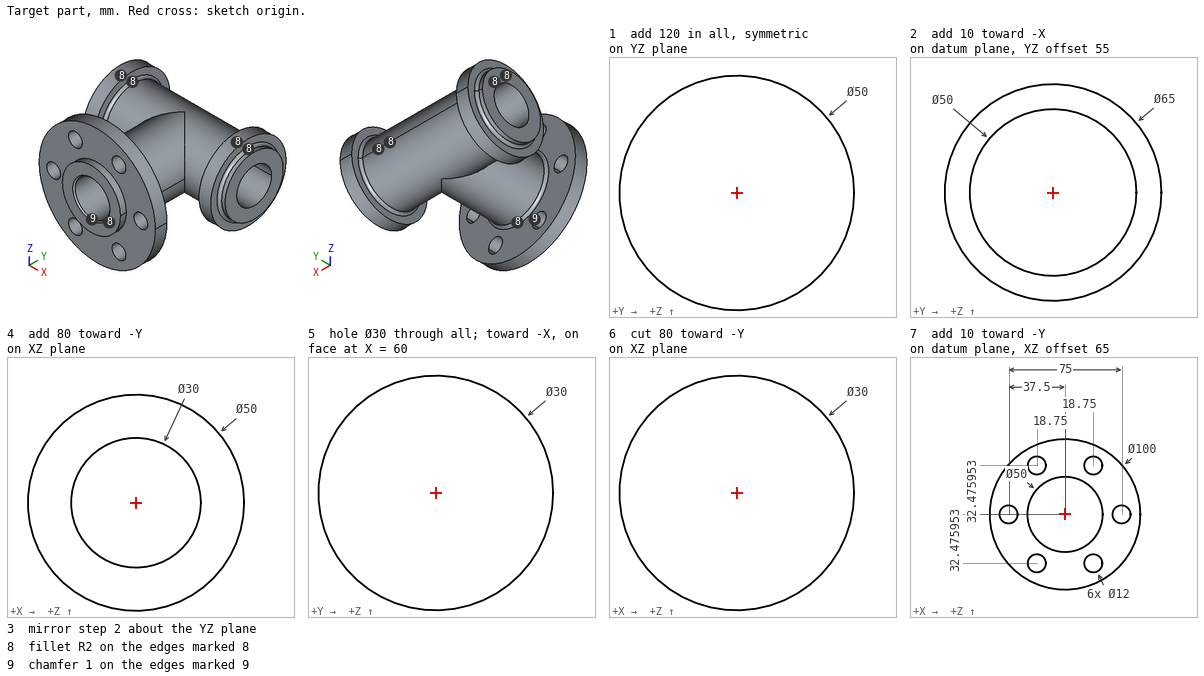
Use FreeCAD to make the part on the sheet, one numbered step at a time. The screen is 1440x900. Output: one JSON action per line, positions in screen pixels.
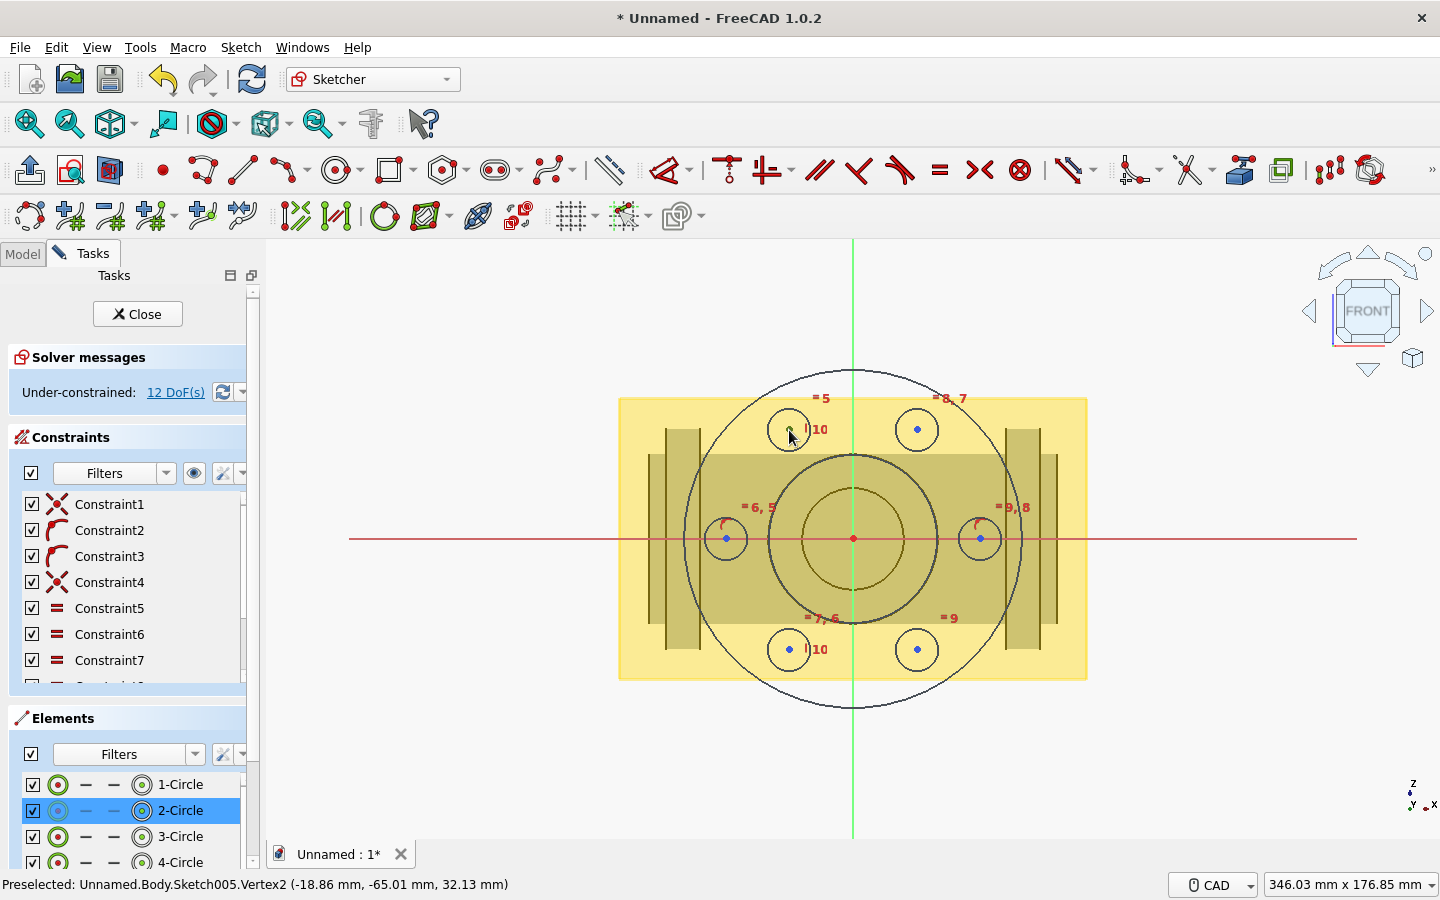
{"action": "left_click", "coordinate": [917, 430]}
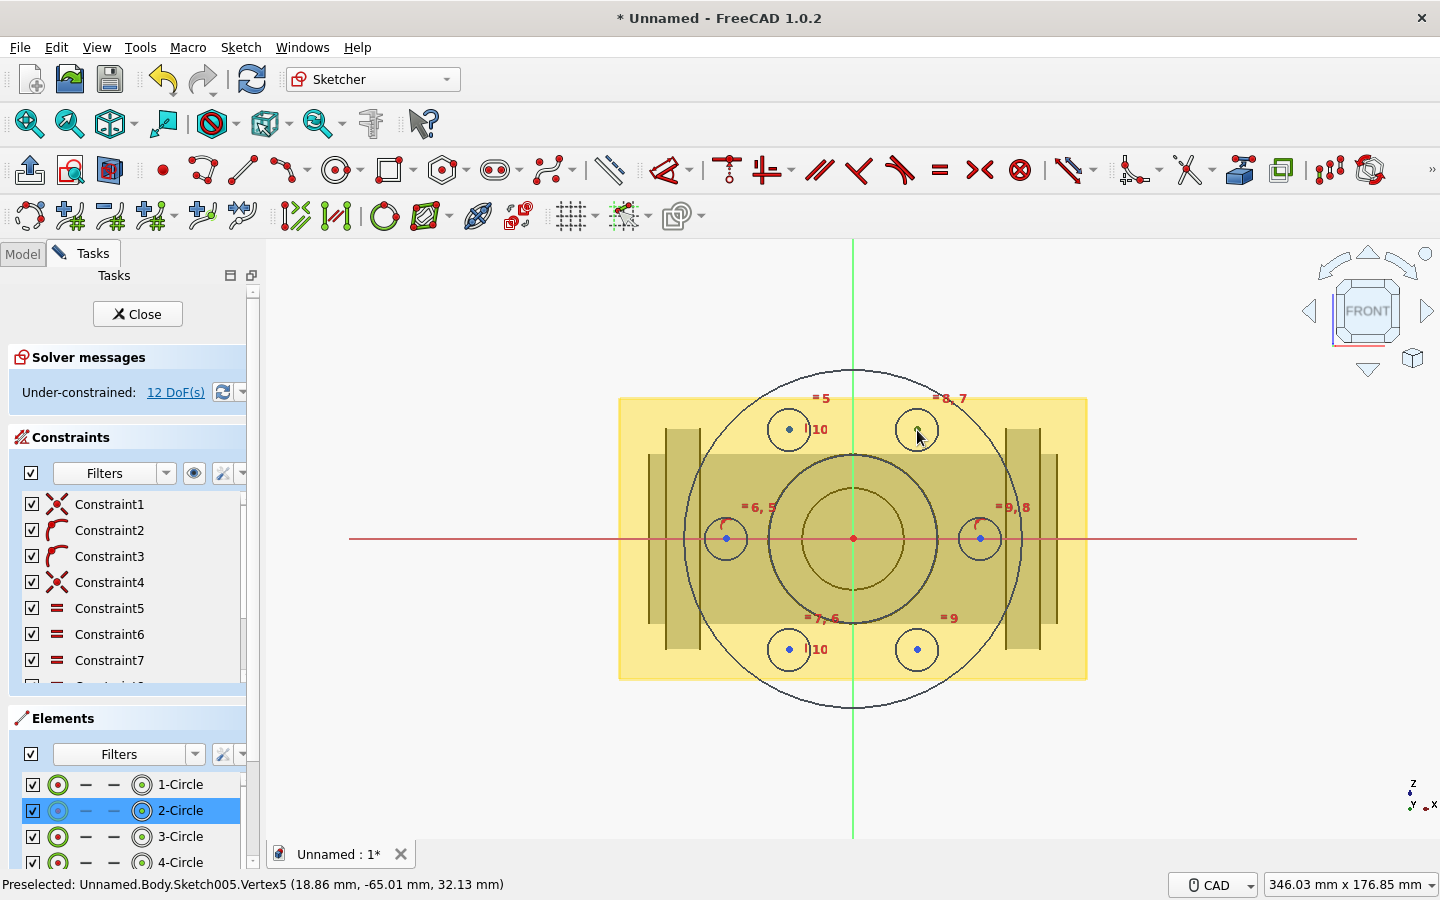
{"action": "left_click", "coordinate": [794, 170]}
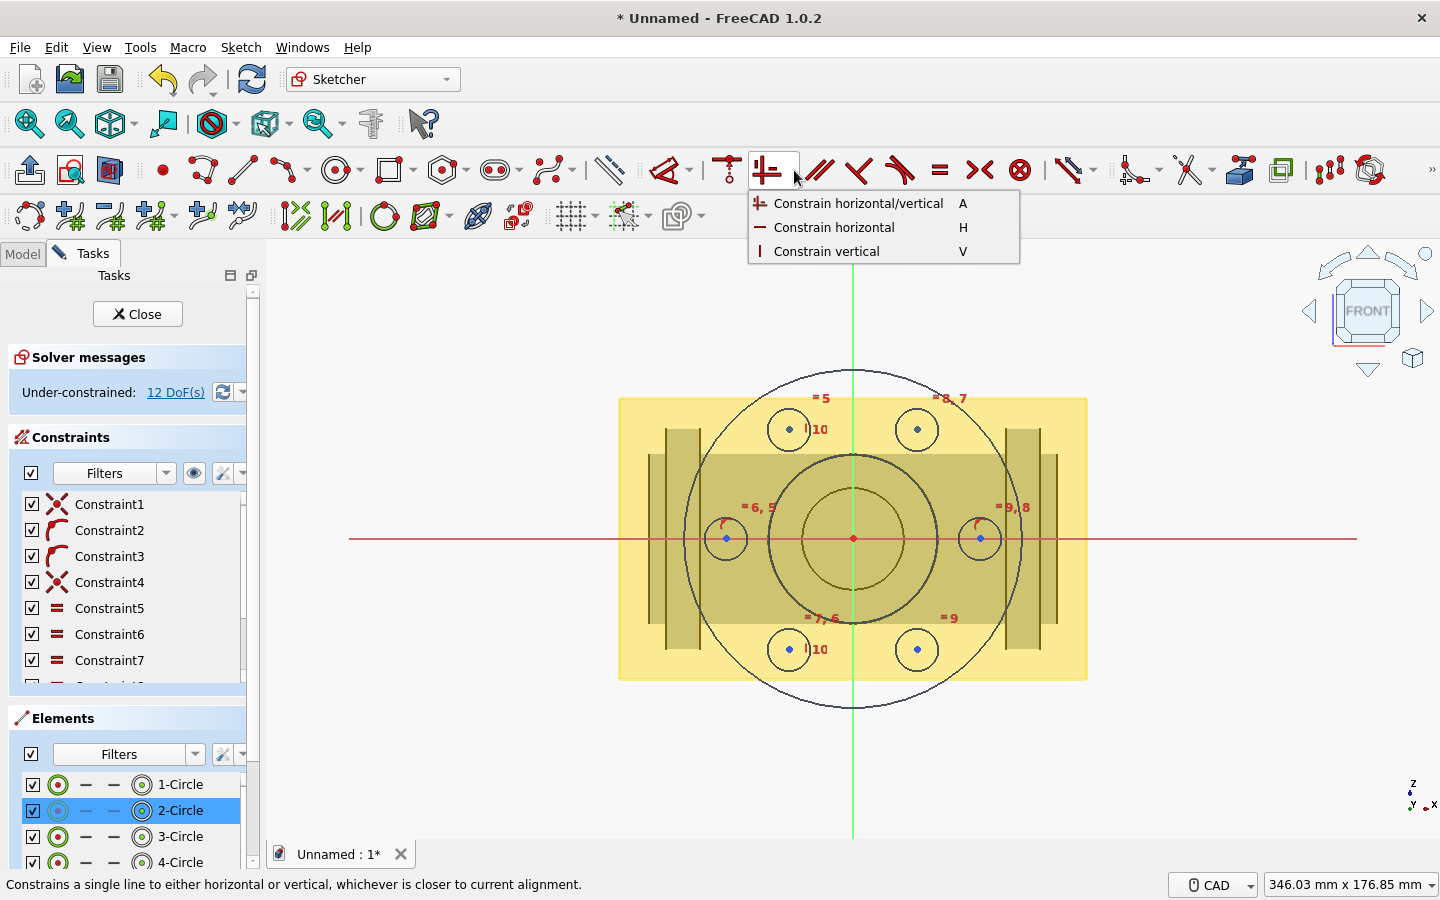
{"action": "left_click", "coordinate": [884, 227]}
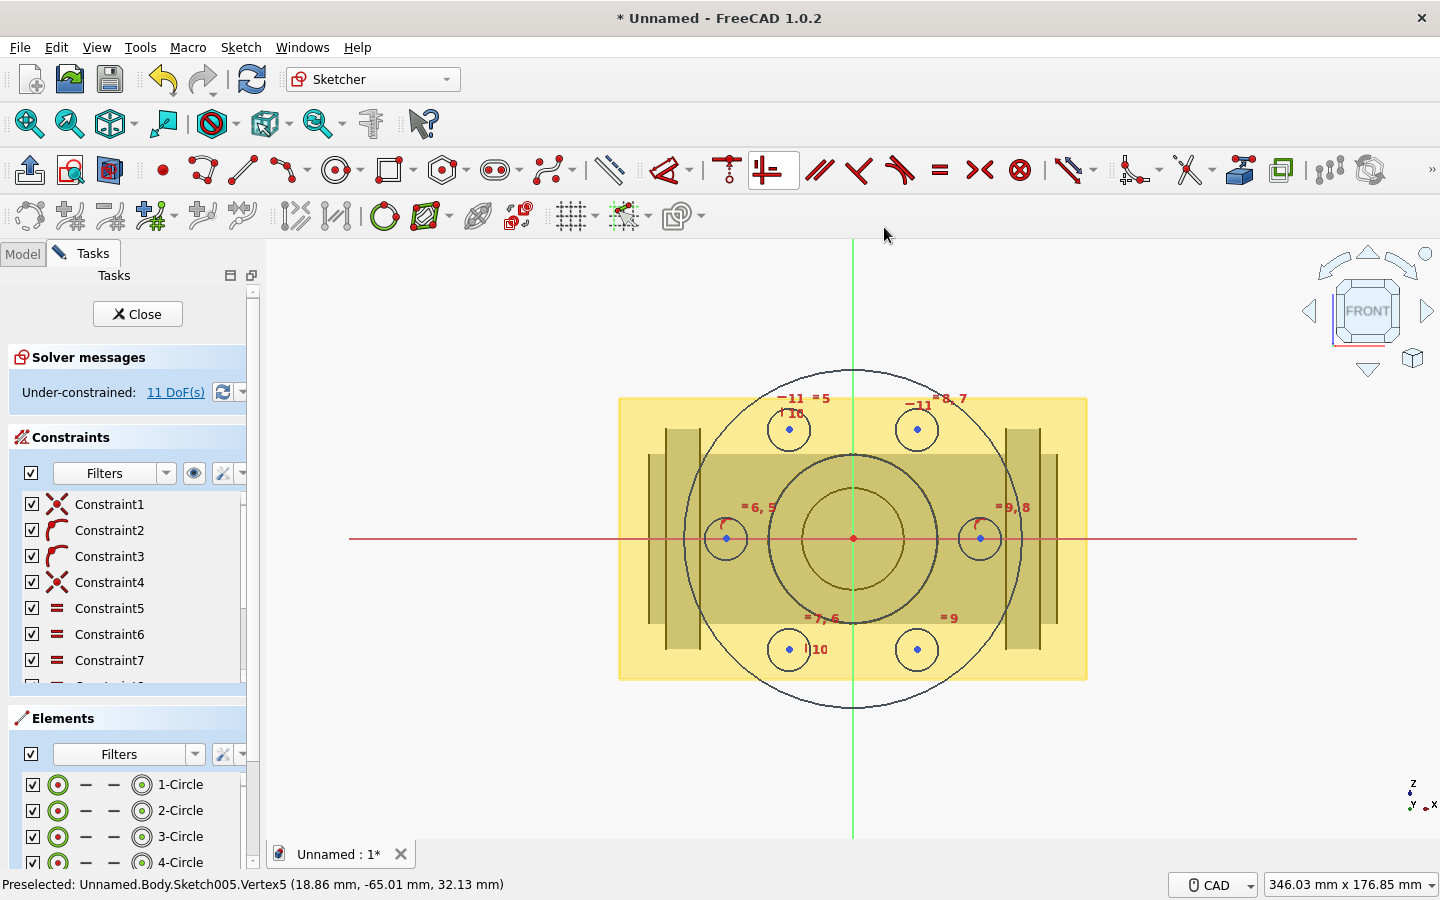
{"action": "left_click", "coordinate": [917, 430]}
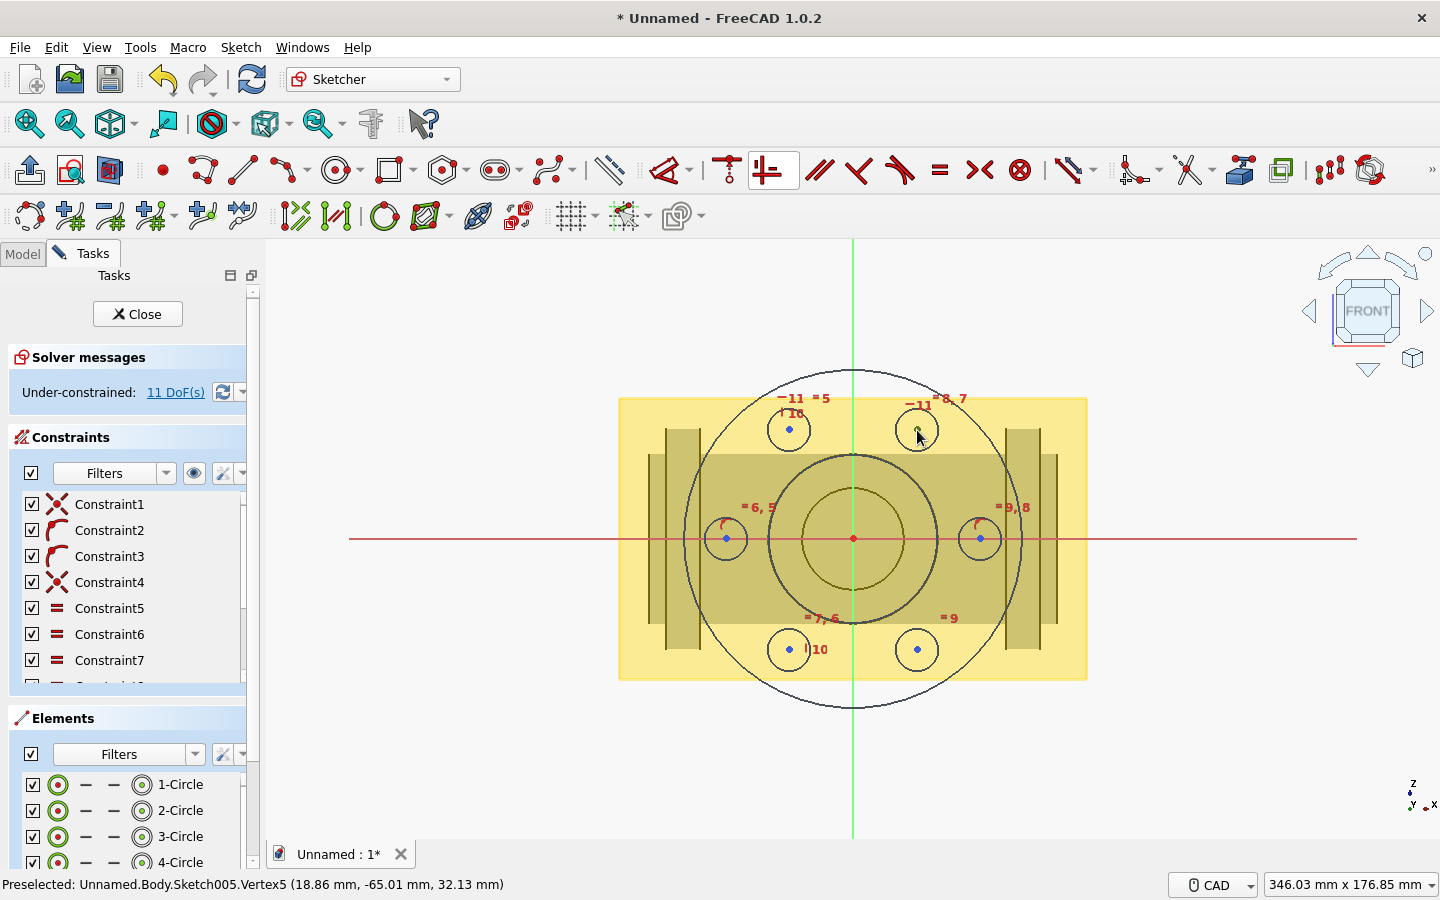
{"action": "left_click", "coordinate": [917, 650]}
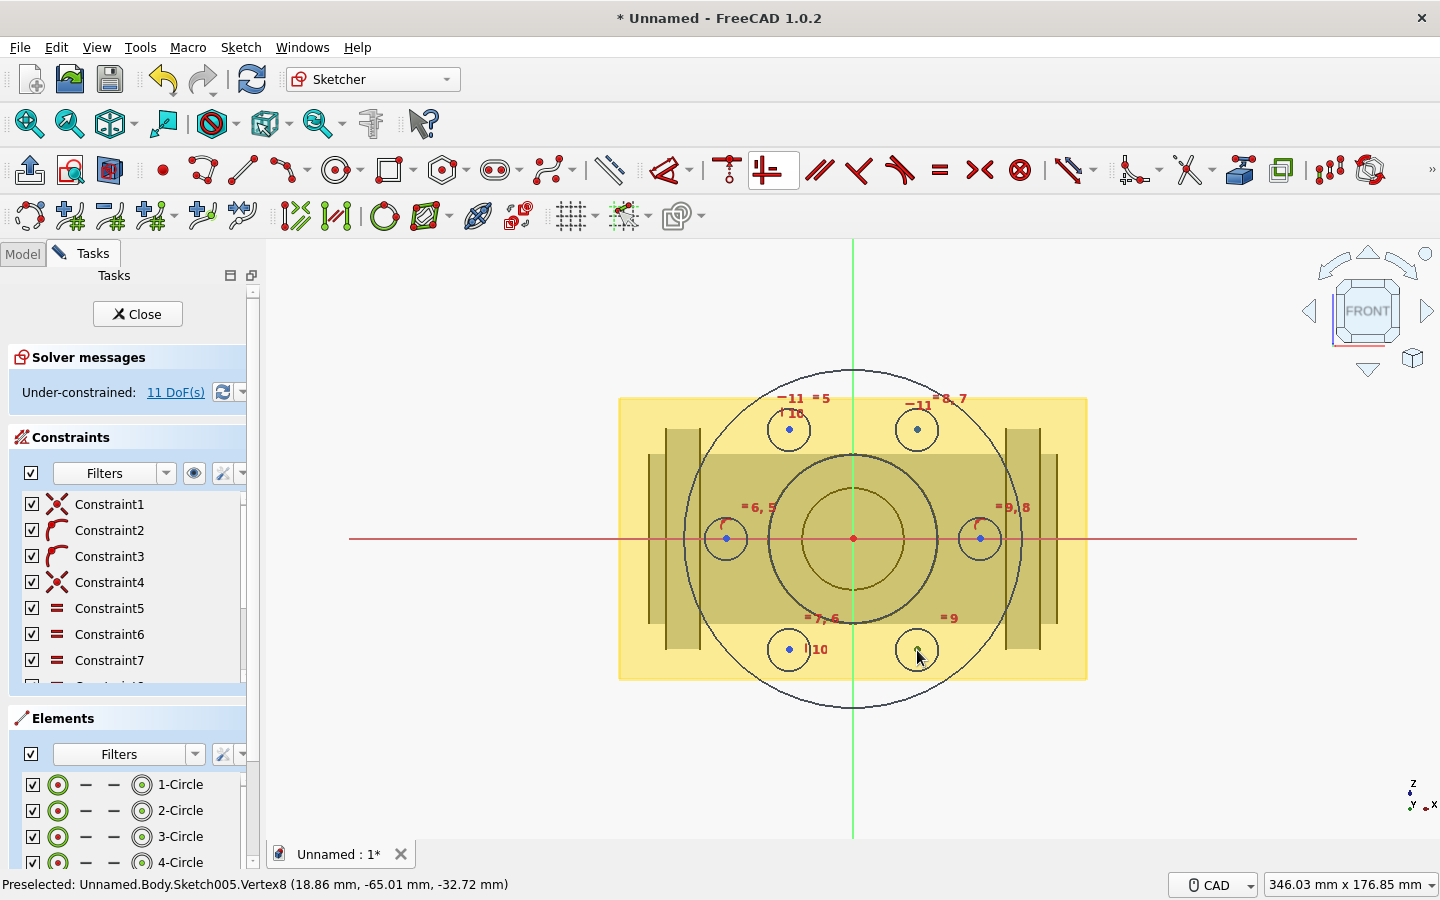
{"action": "key", "text": "v"}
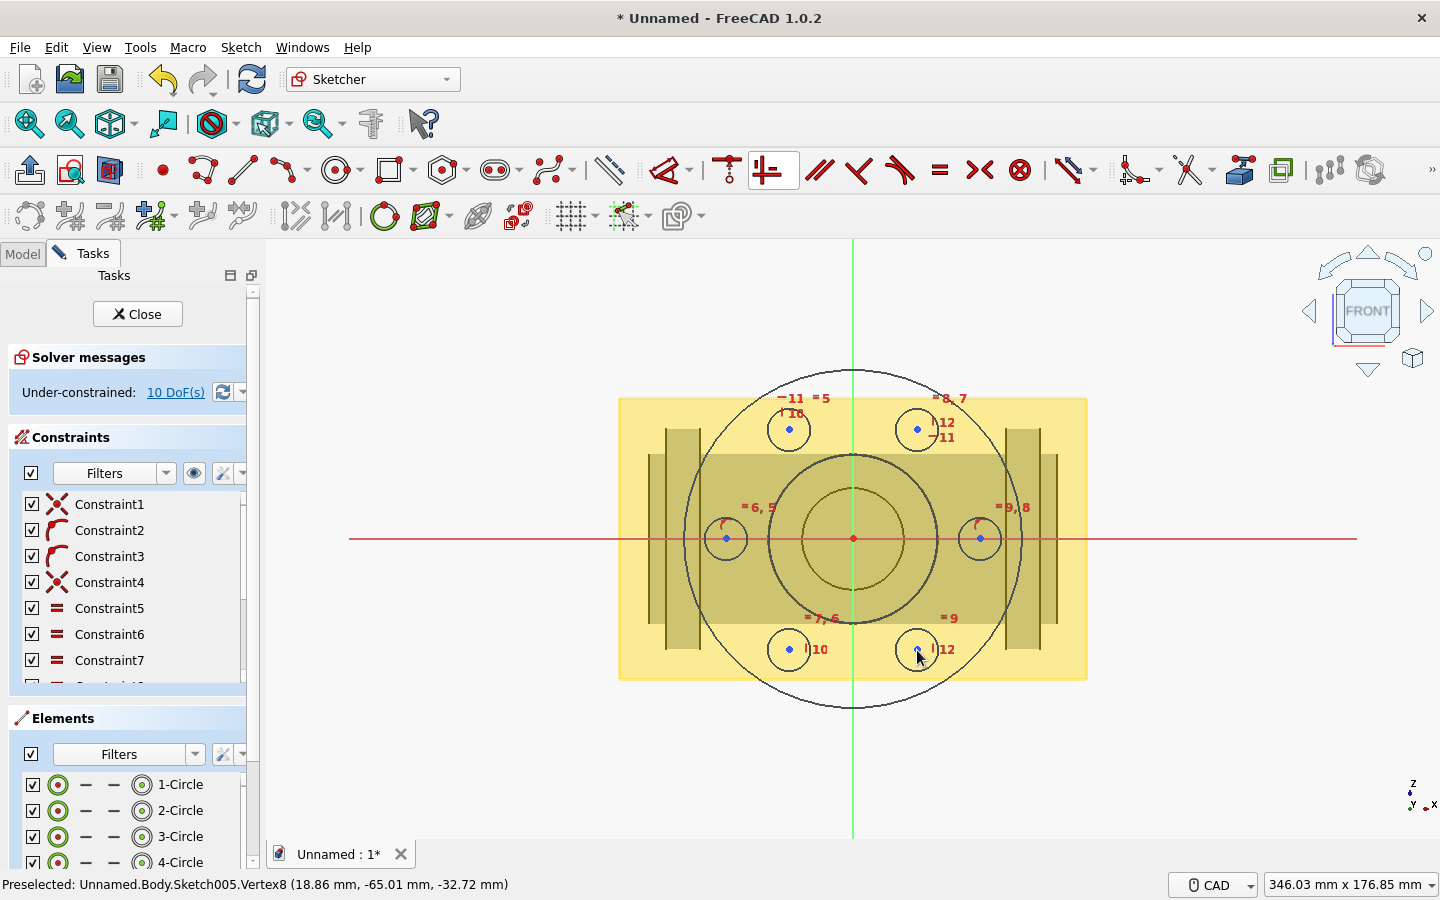
{"action": "left_click", "coordinate": [789, 650]}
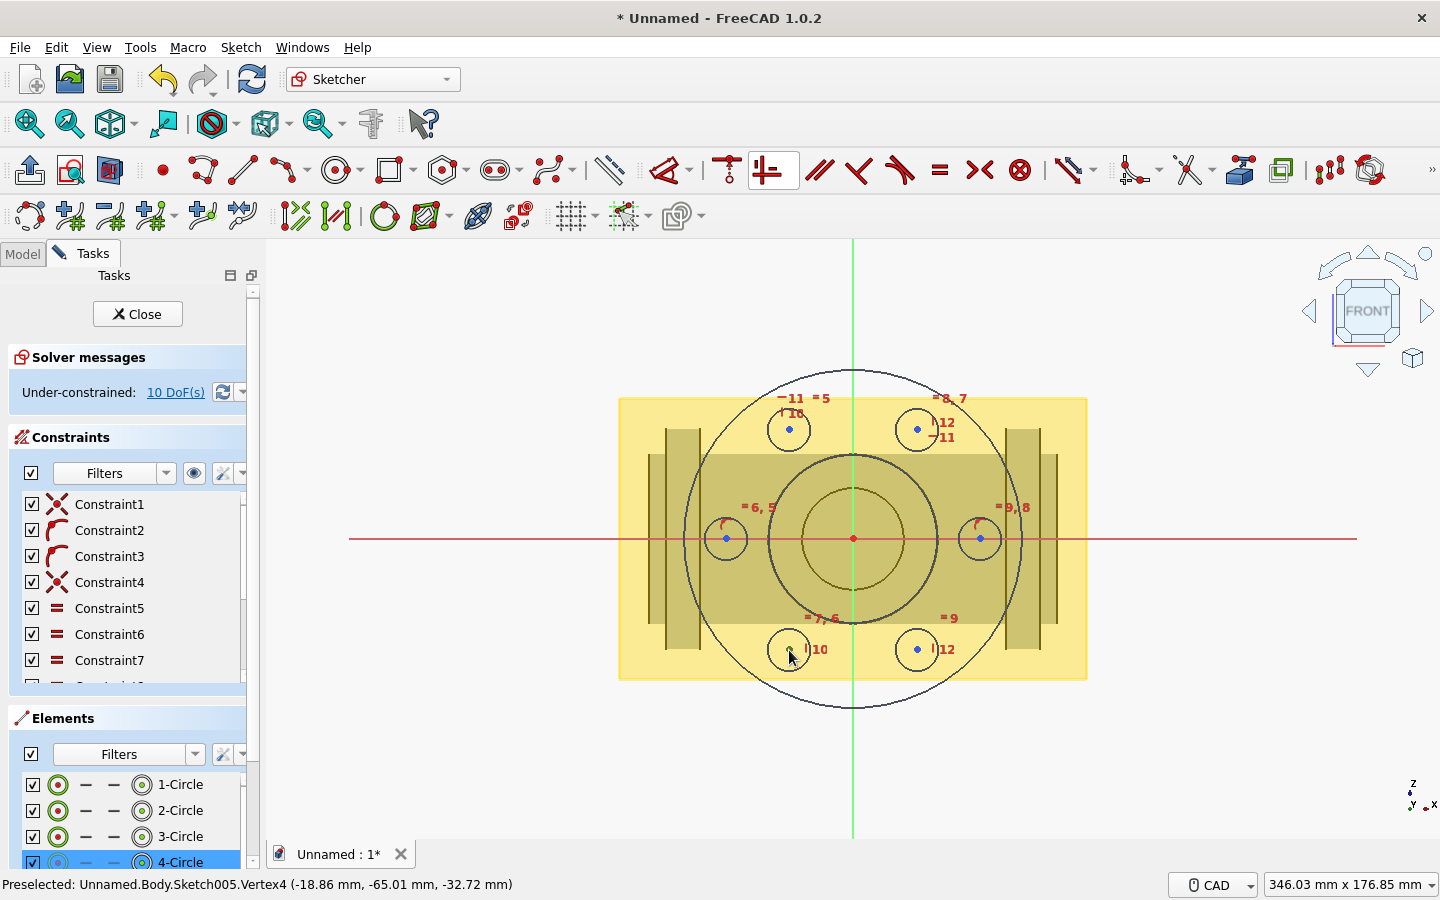
{"action": "left_click", "coordinate": [917, 650]}